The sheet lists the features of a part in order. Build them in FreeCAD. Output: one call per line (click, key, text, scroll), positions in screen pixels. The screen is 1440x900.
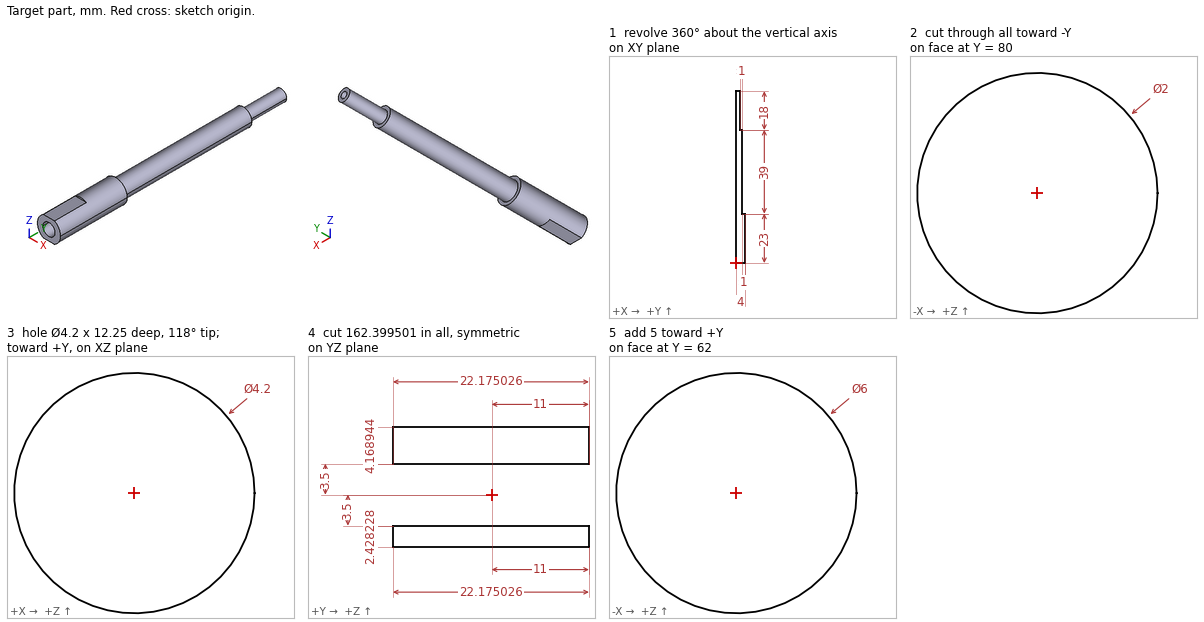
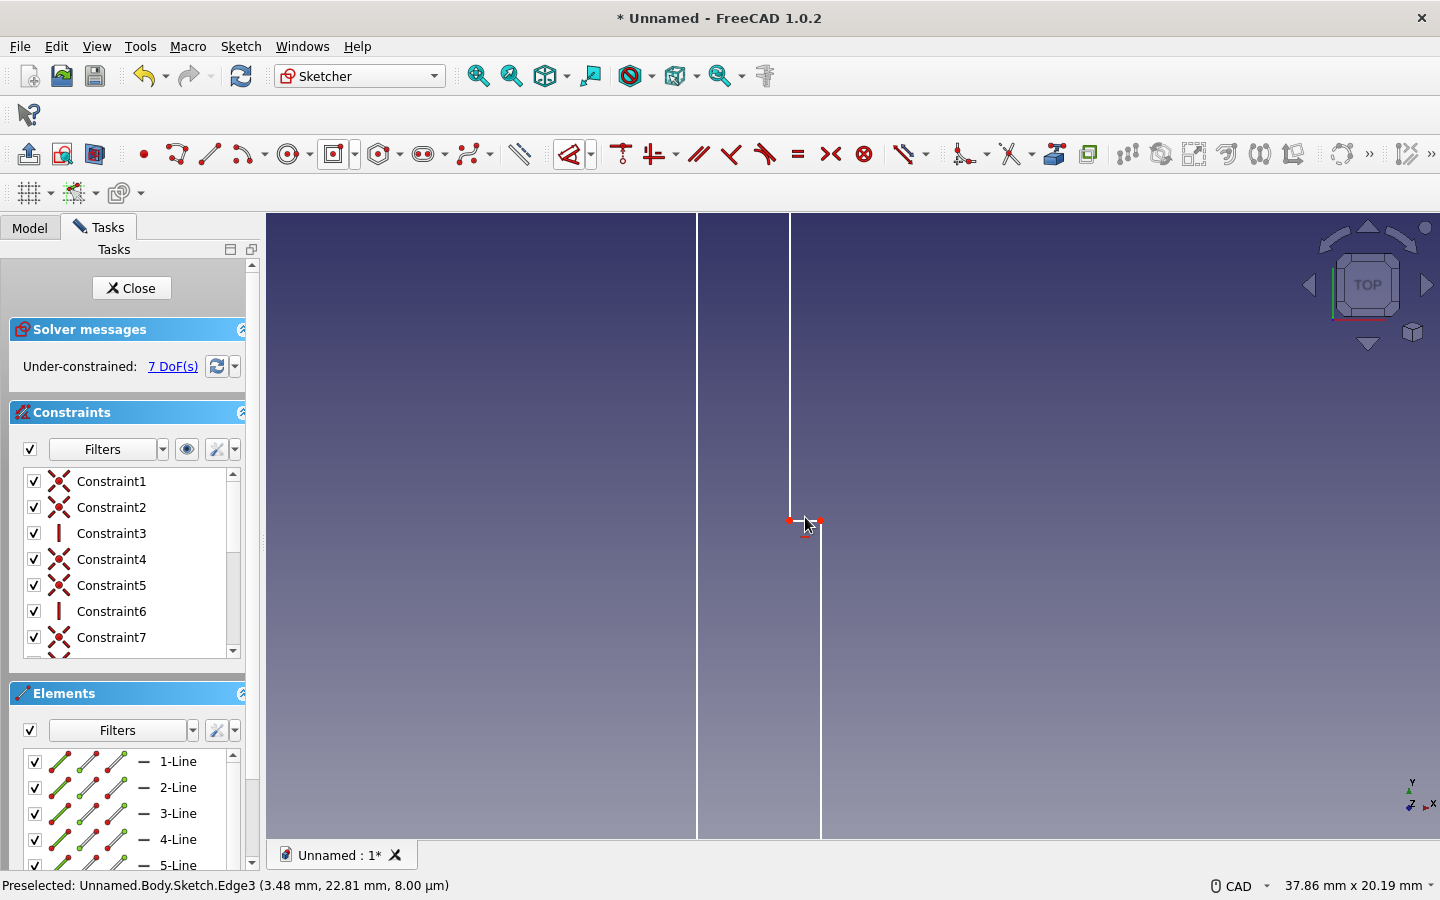
scroll(790, 633, down, 9)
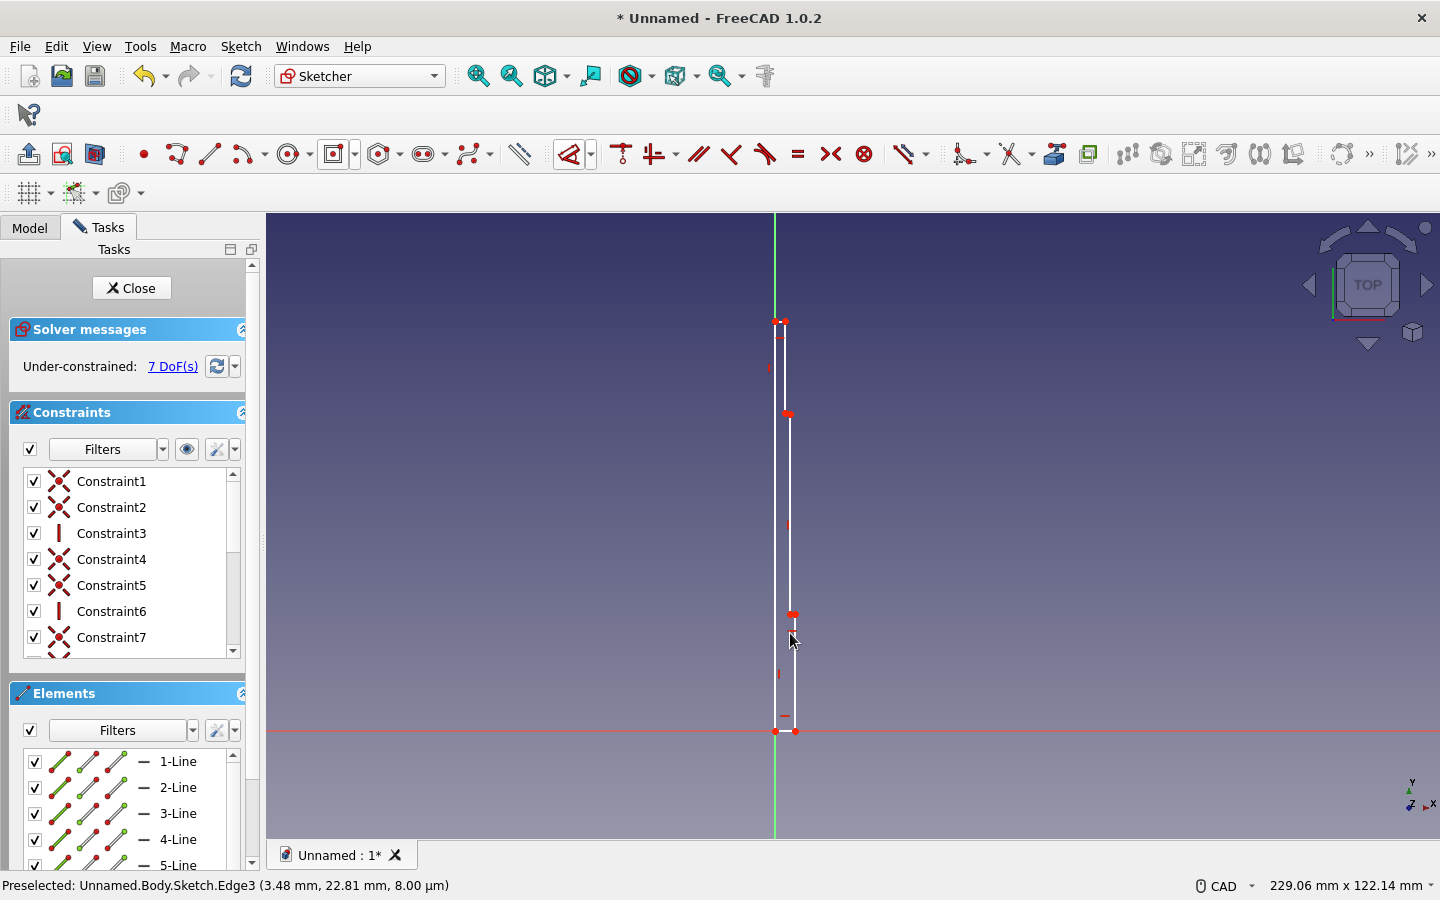
scroll(789, 414, up, 11)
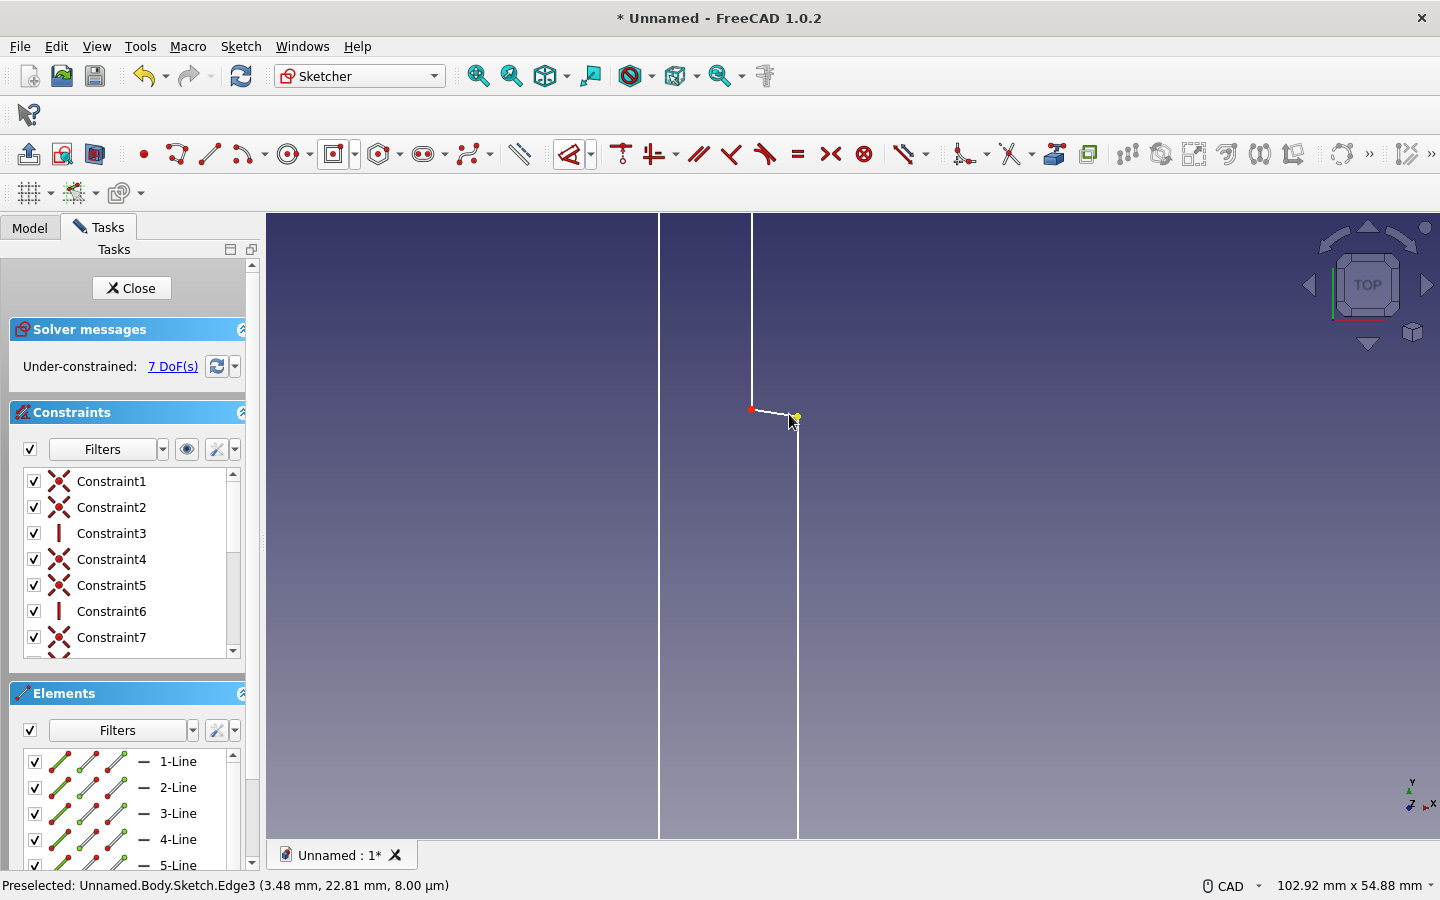
click(784, 414)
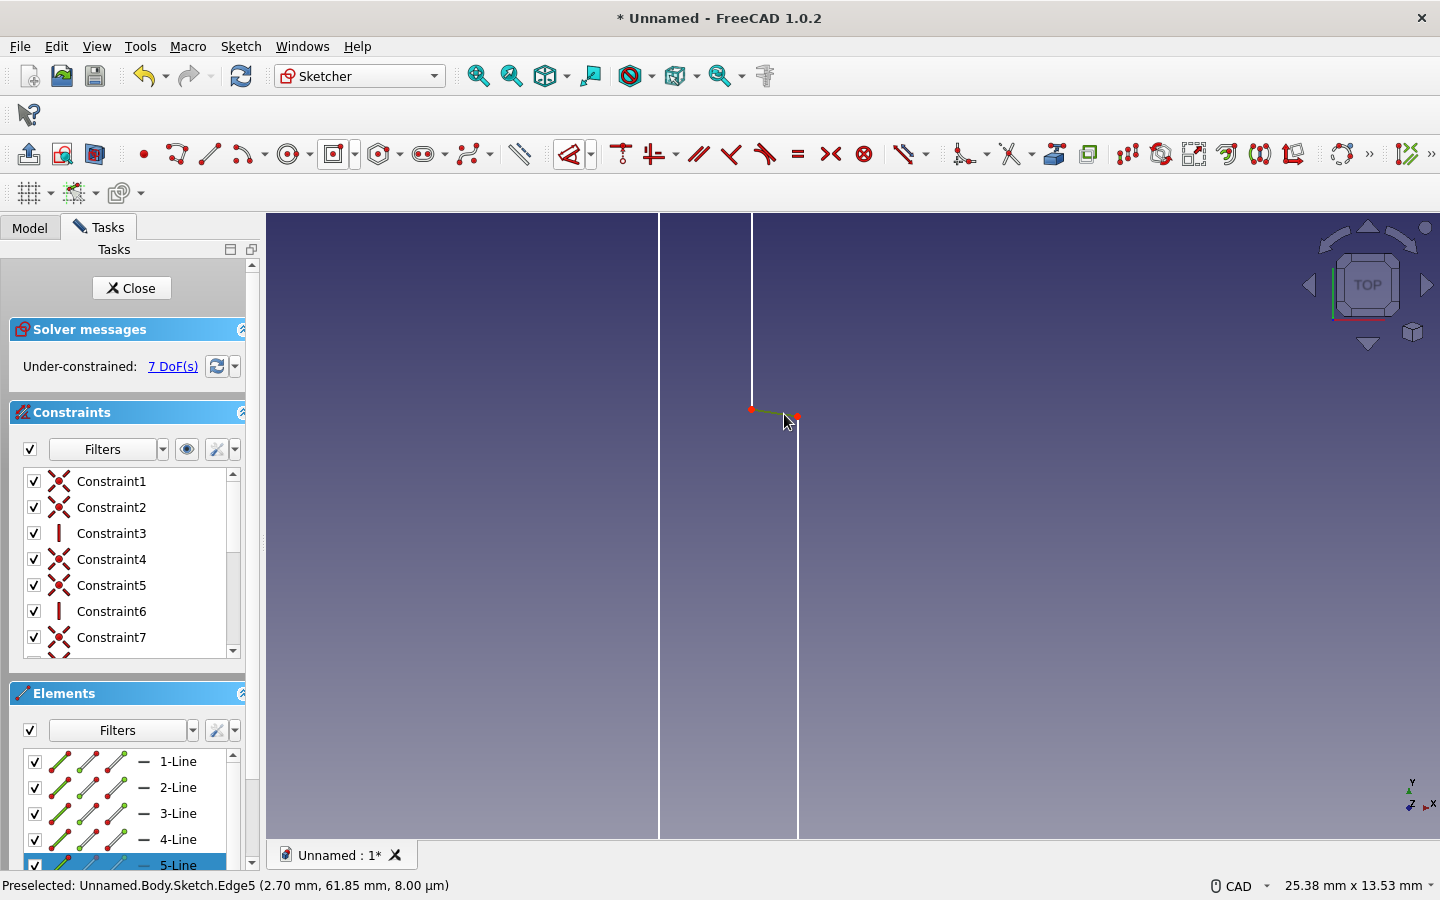
key(h)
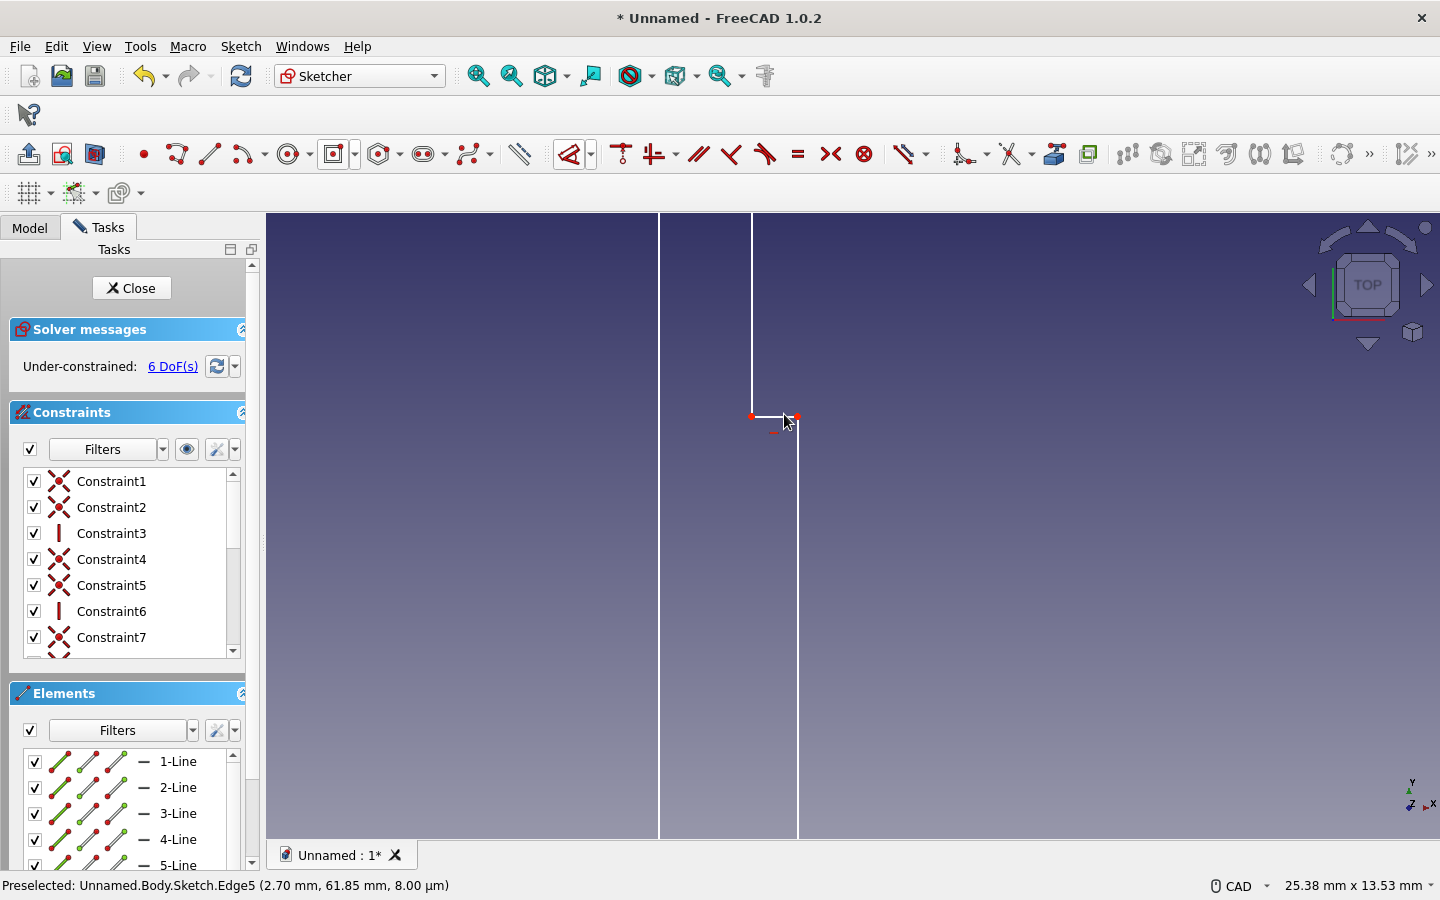
scroll(789, 414, down, 11)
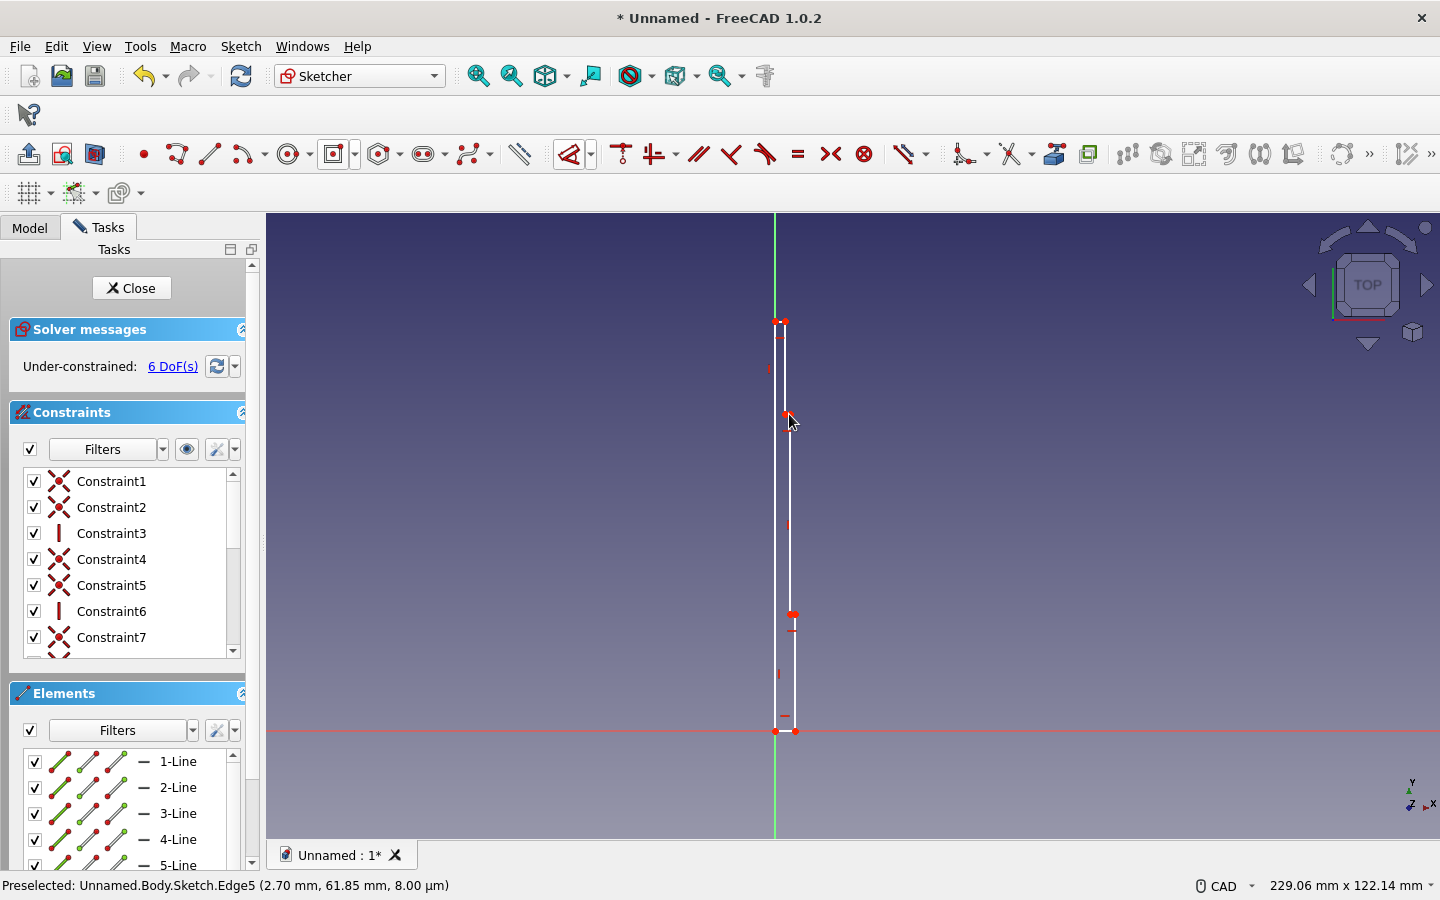
scroll(781, 731, up, 5)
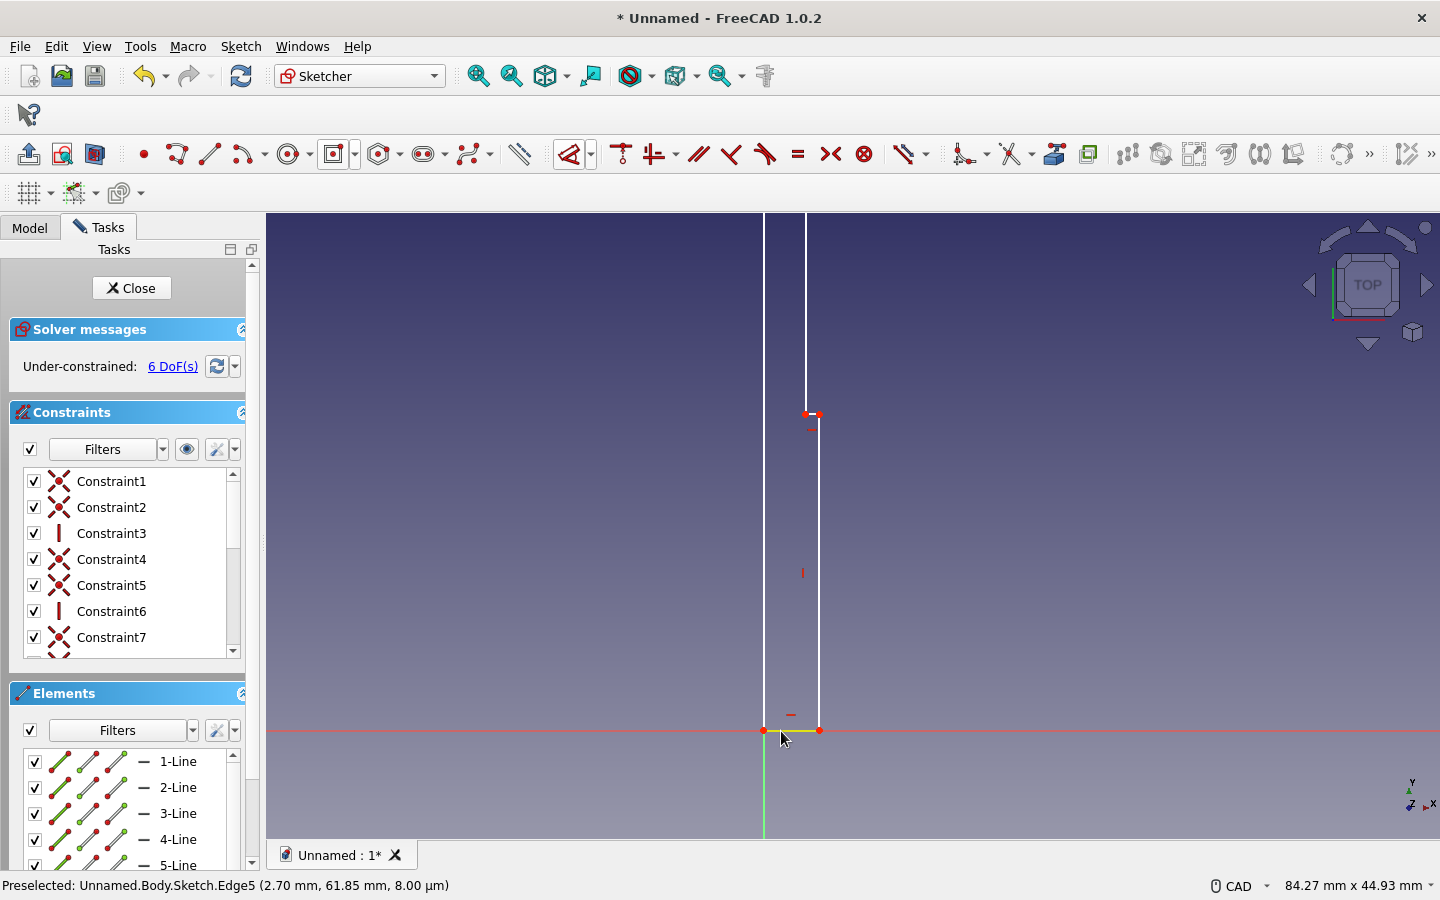
click(781, 731)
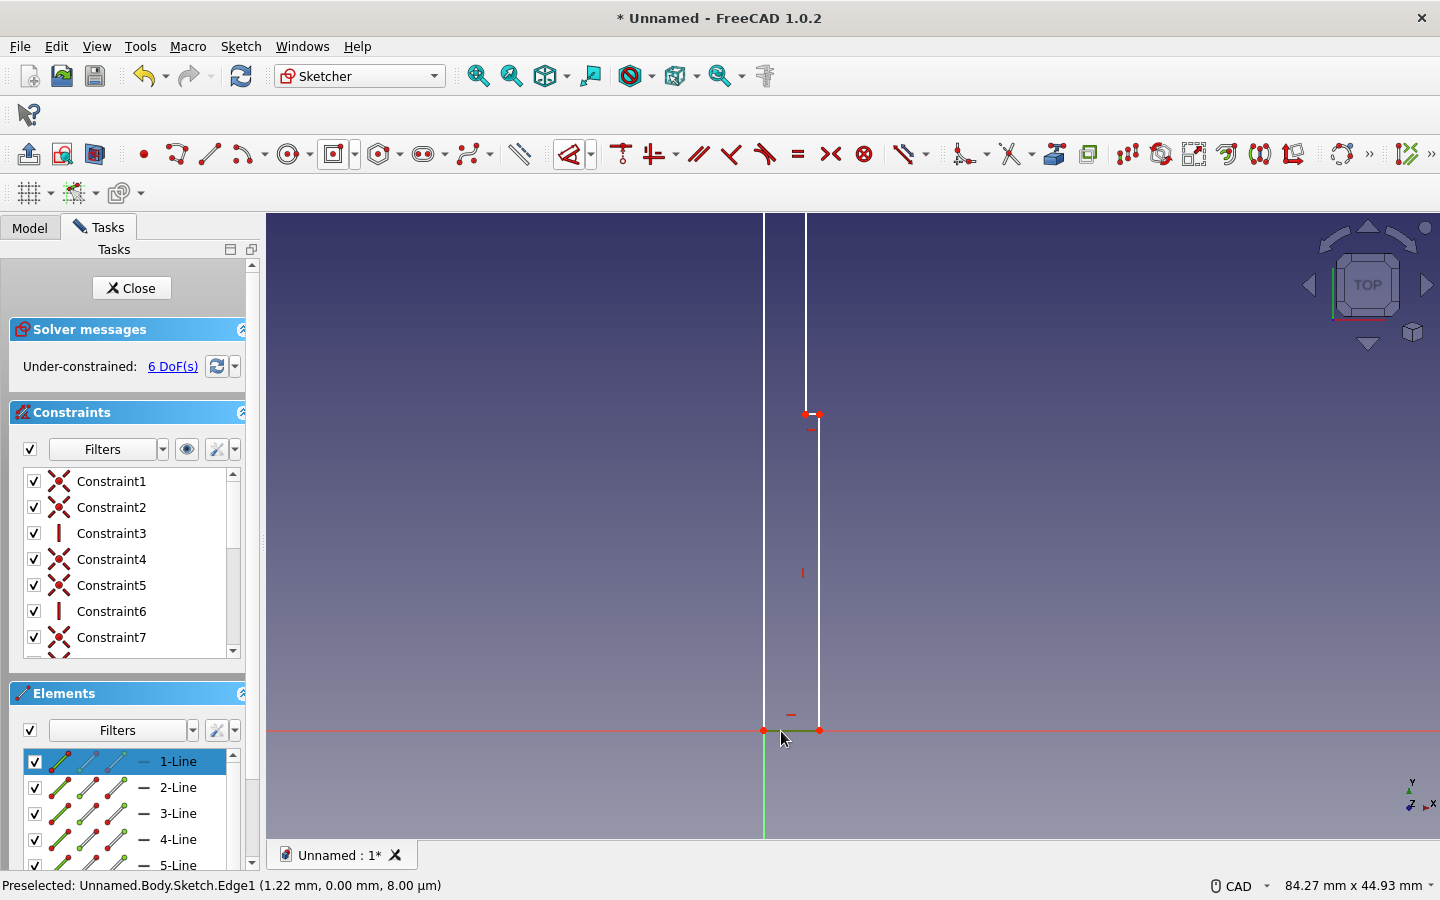
key(l)